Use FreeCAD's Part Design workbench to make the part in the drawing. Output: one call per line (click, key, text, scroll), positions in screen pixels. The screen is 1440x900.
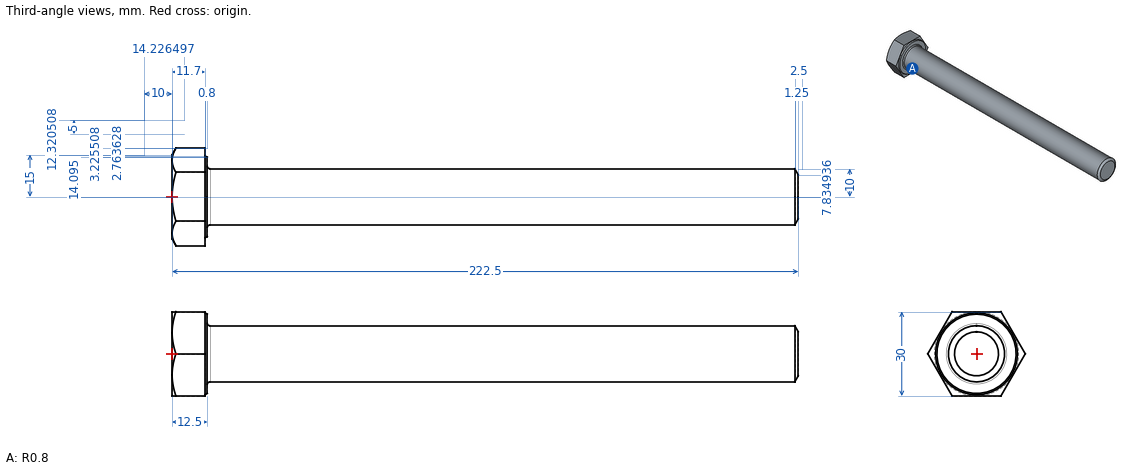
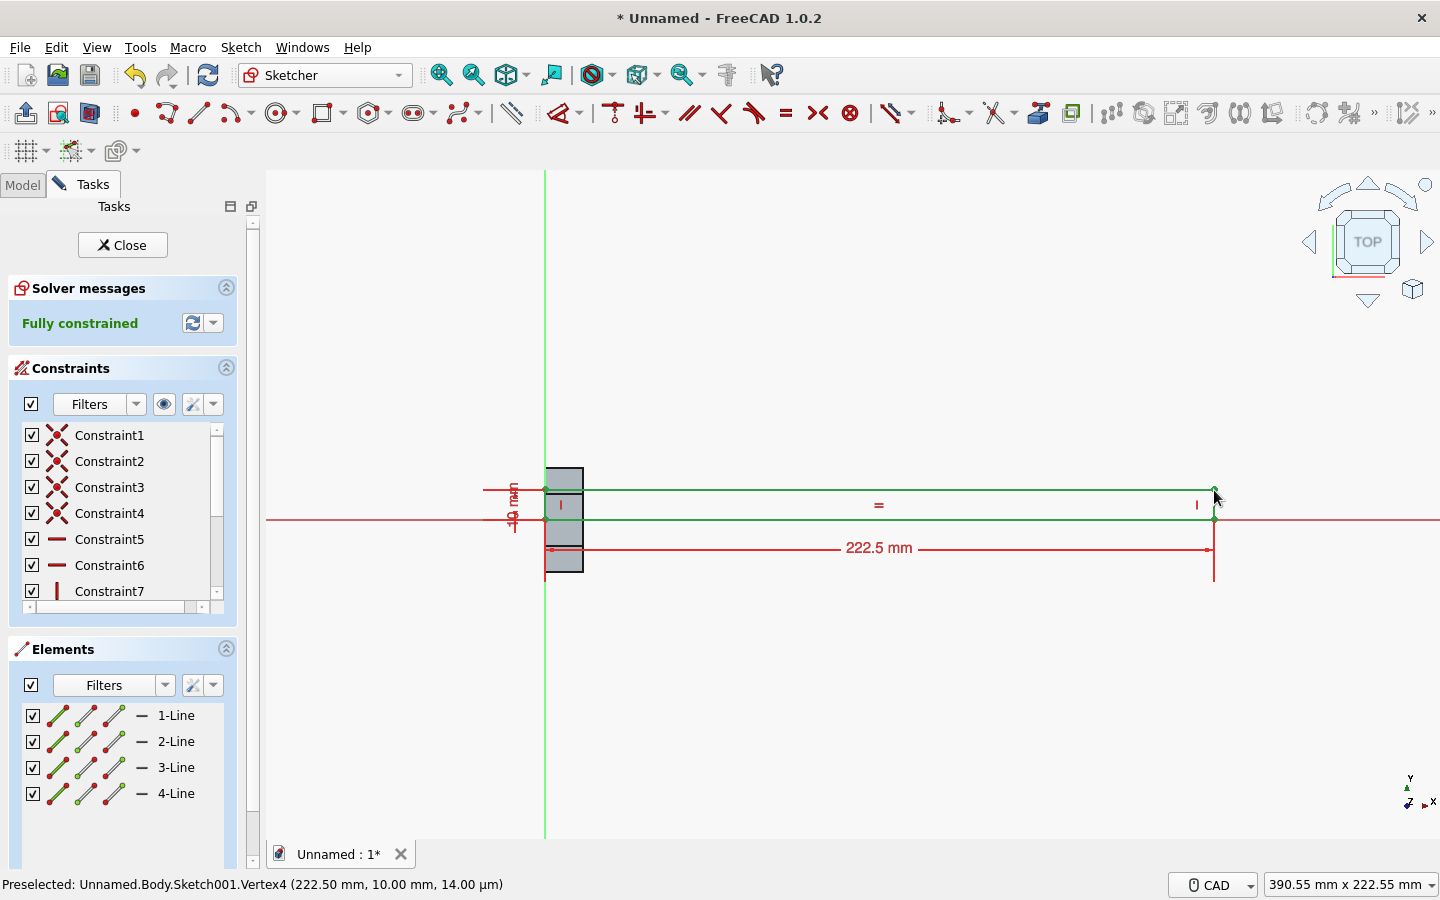
click(123, 245)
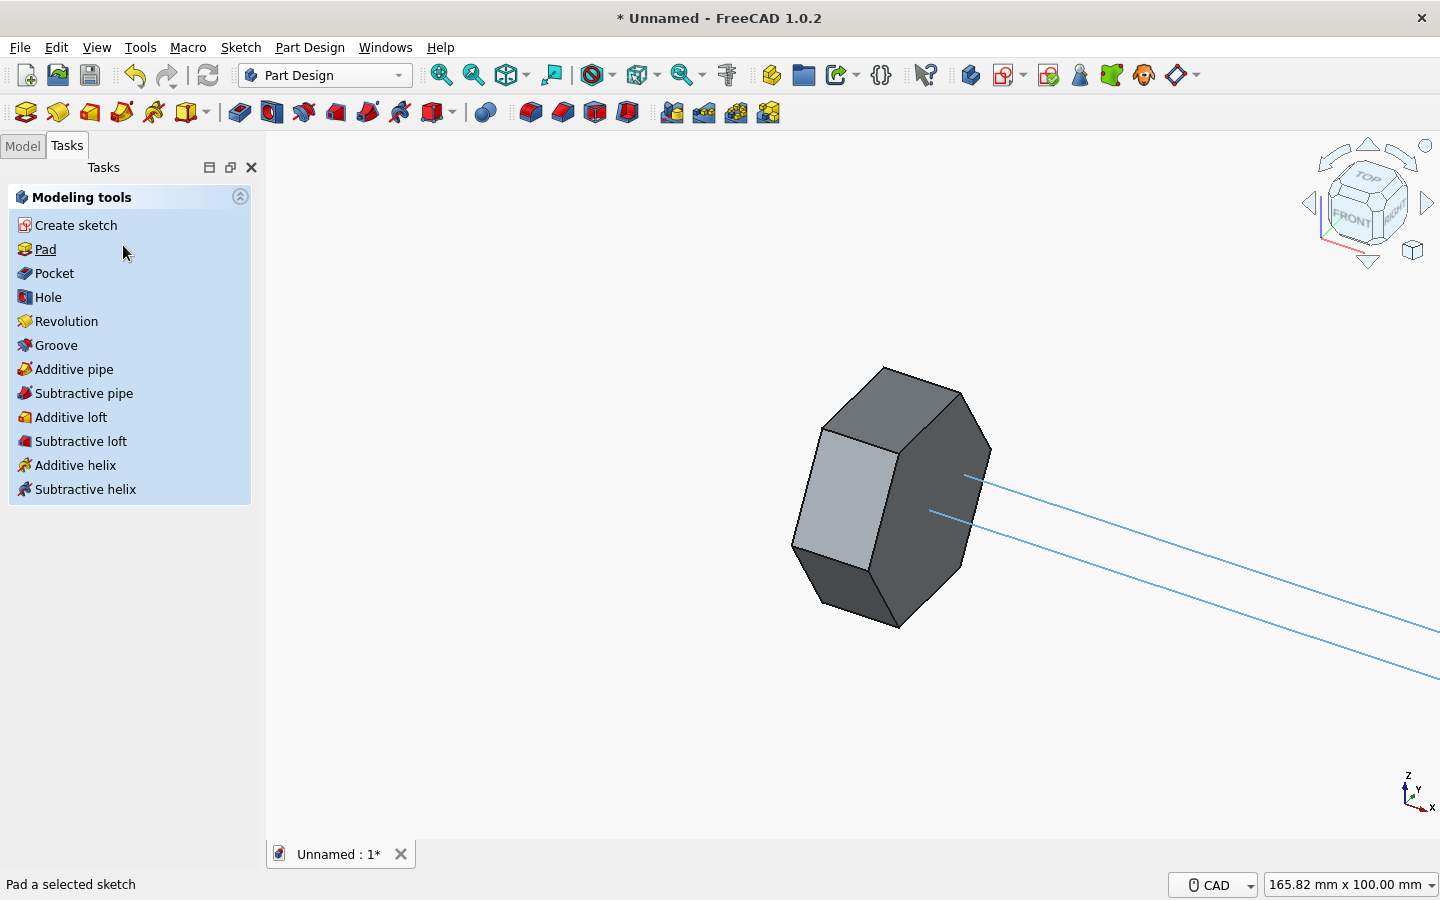
click(58, 112)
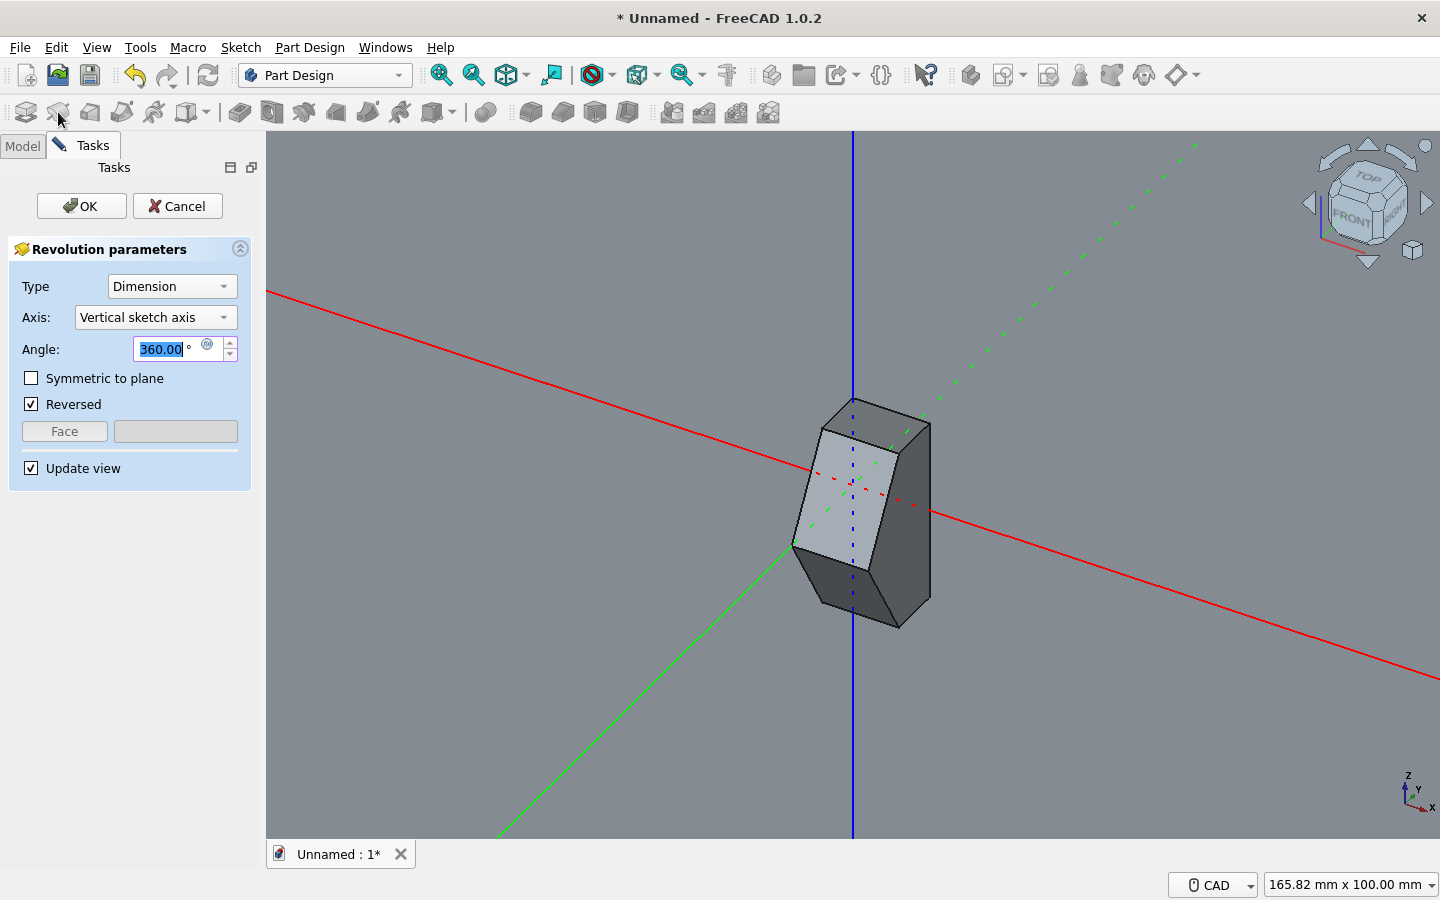
click(156, 318)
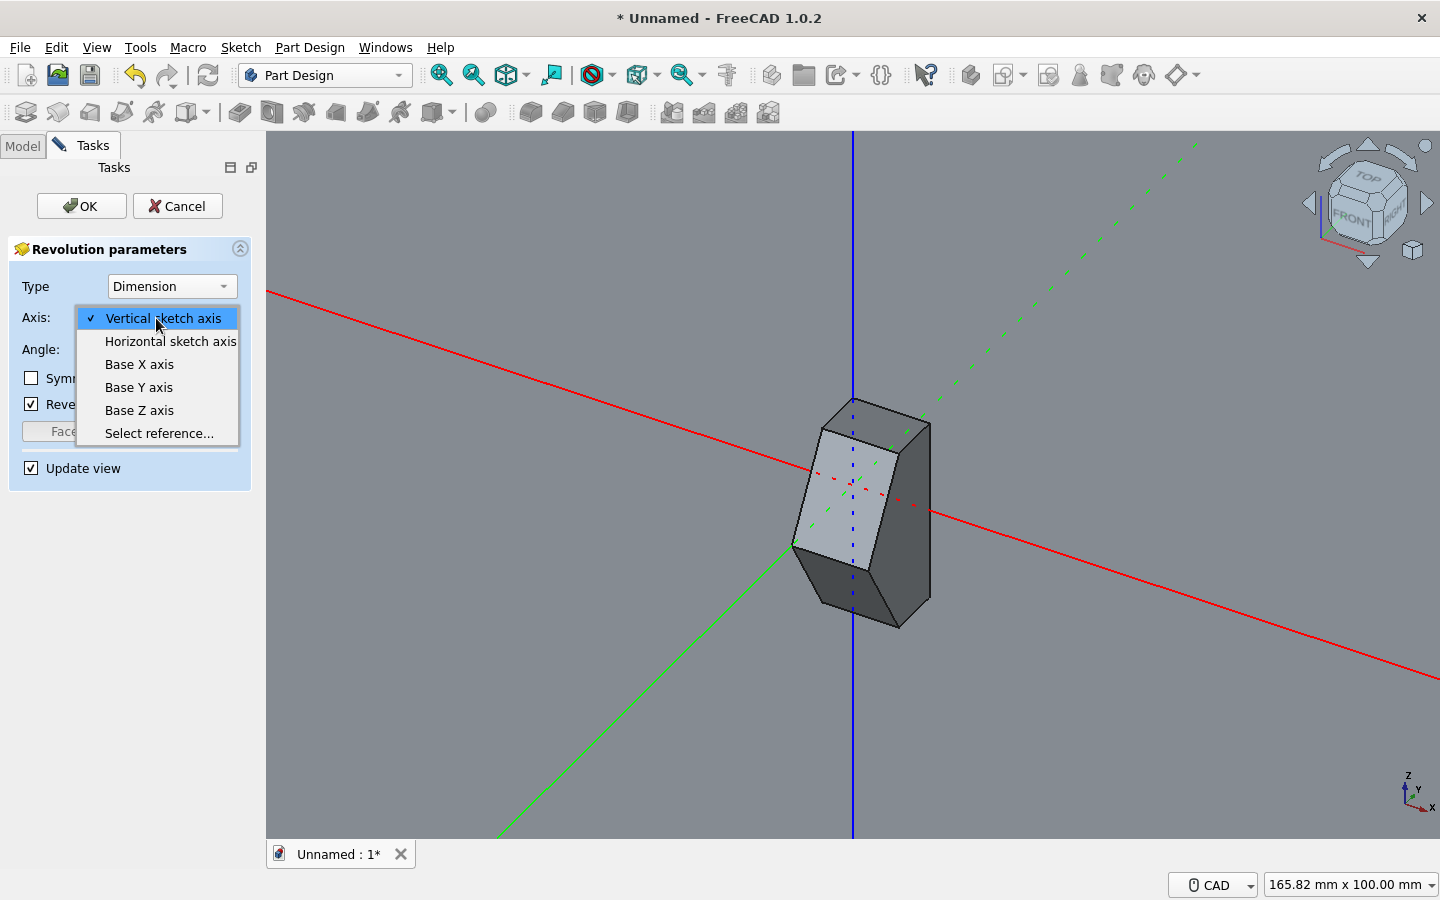
click(156, 342)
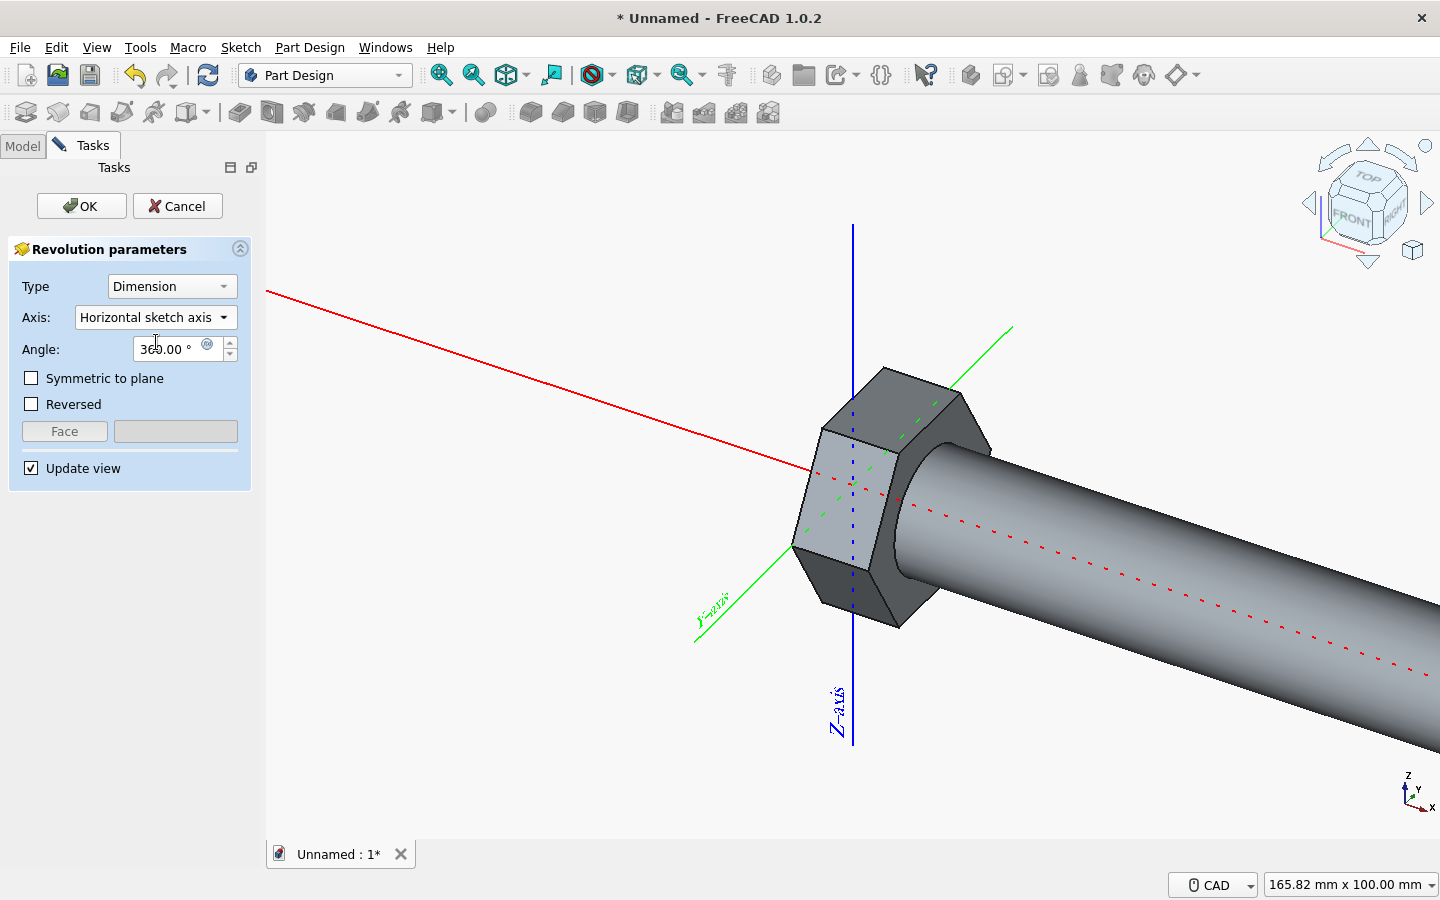
click(82, 206)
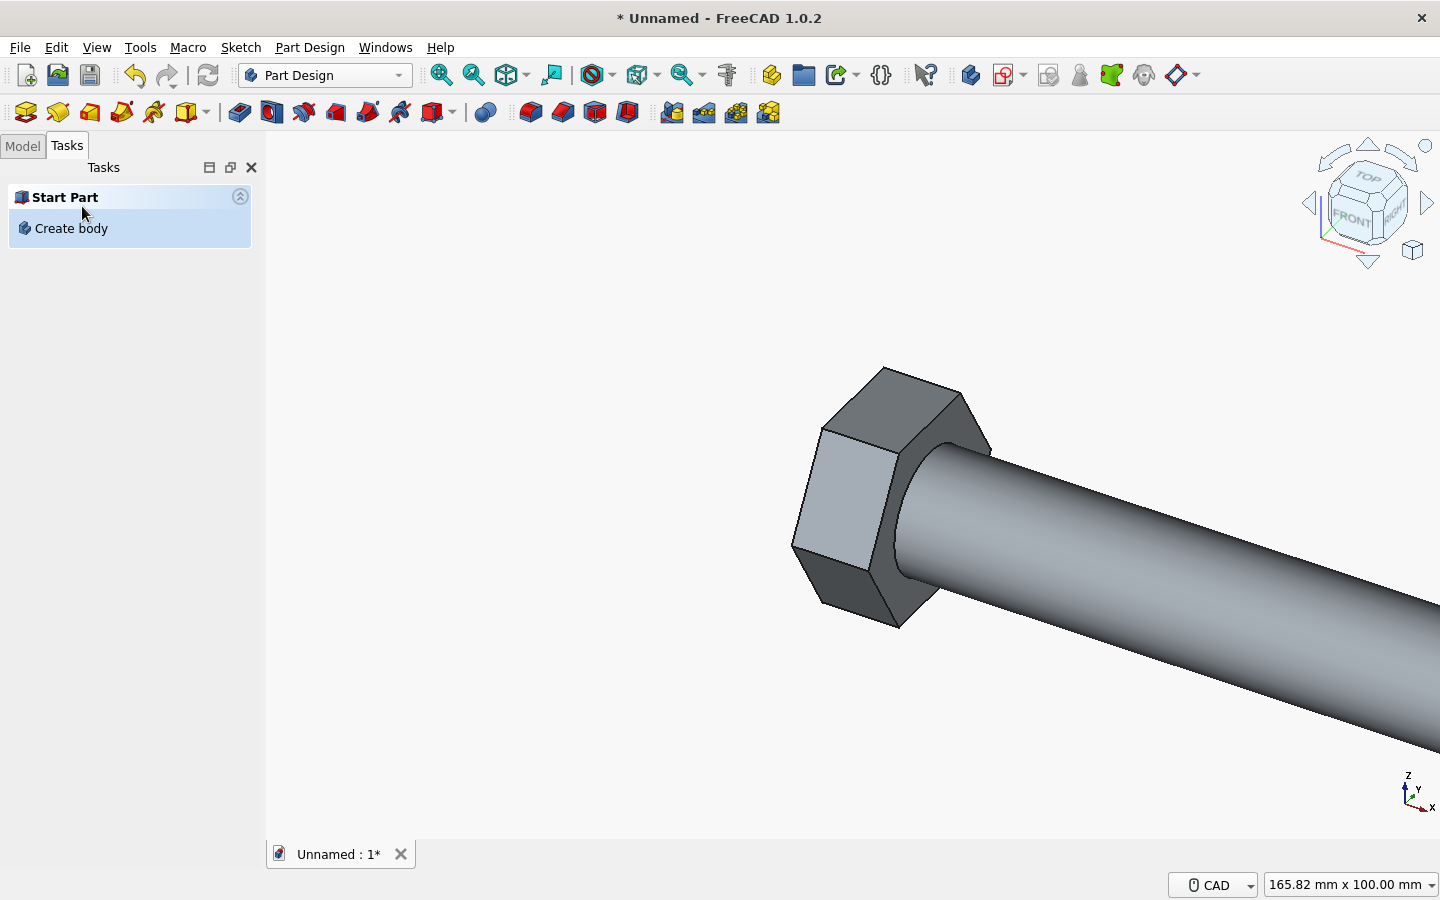
click(442, 76)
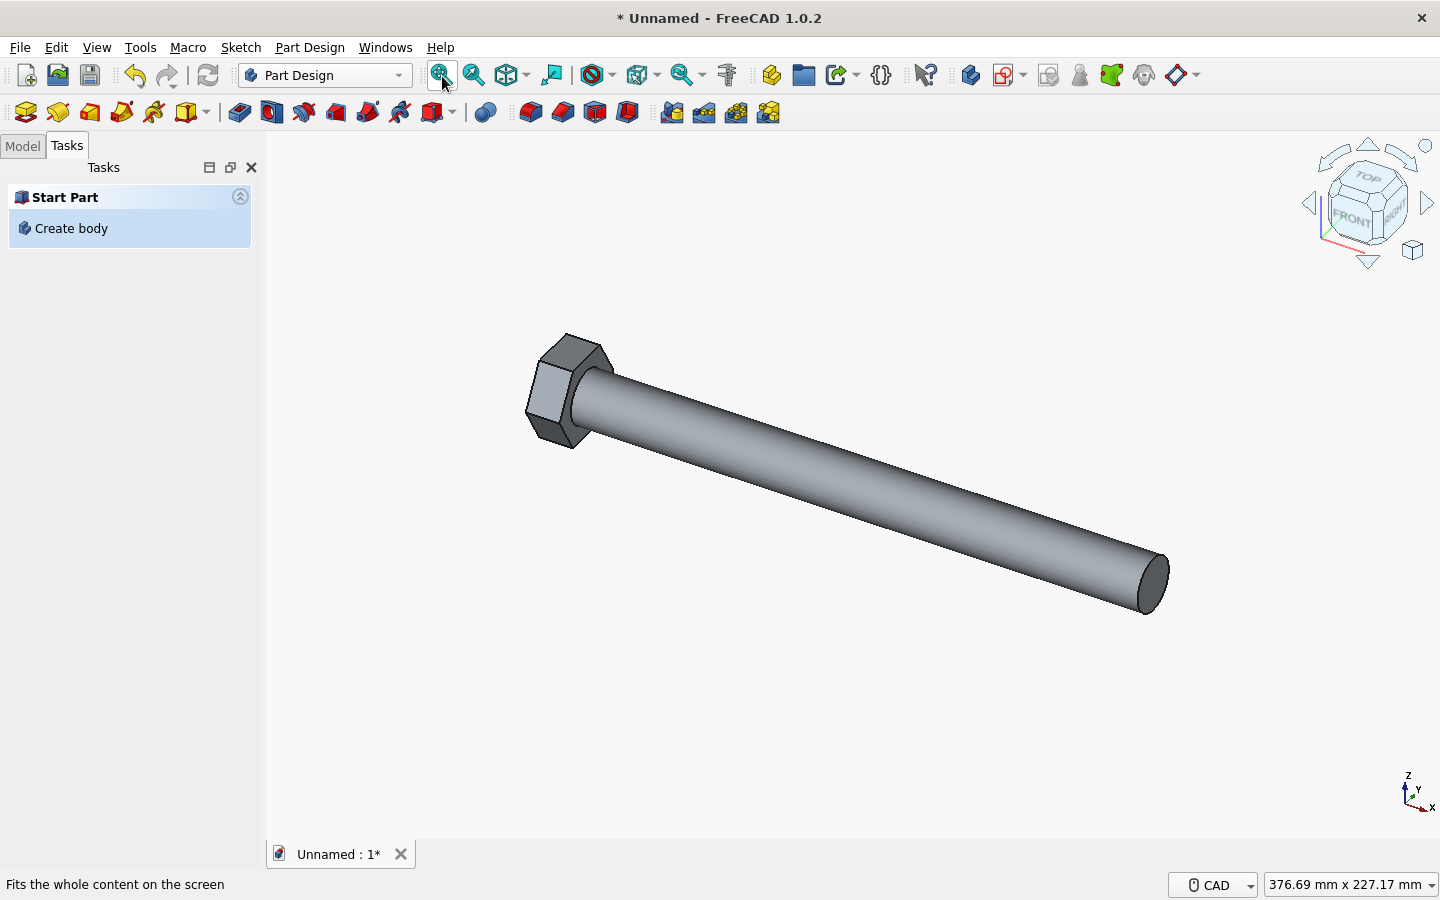
click(1004, 76)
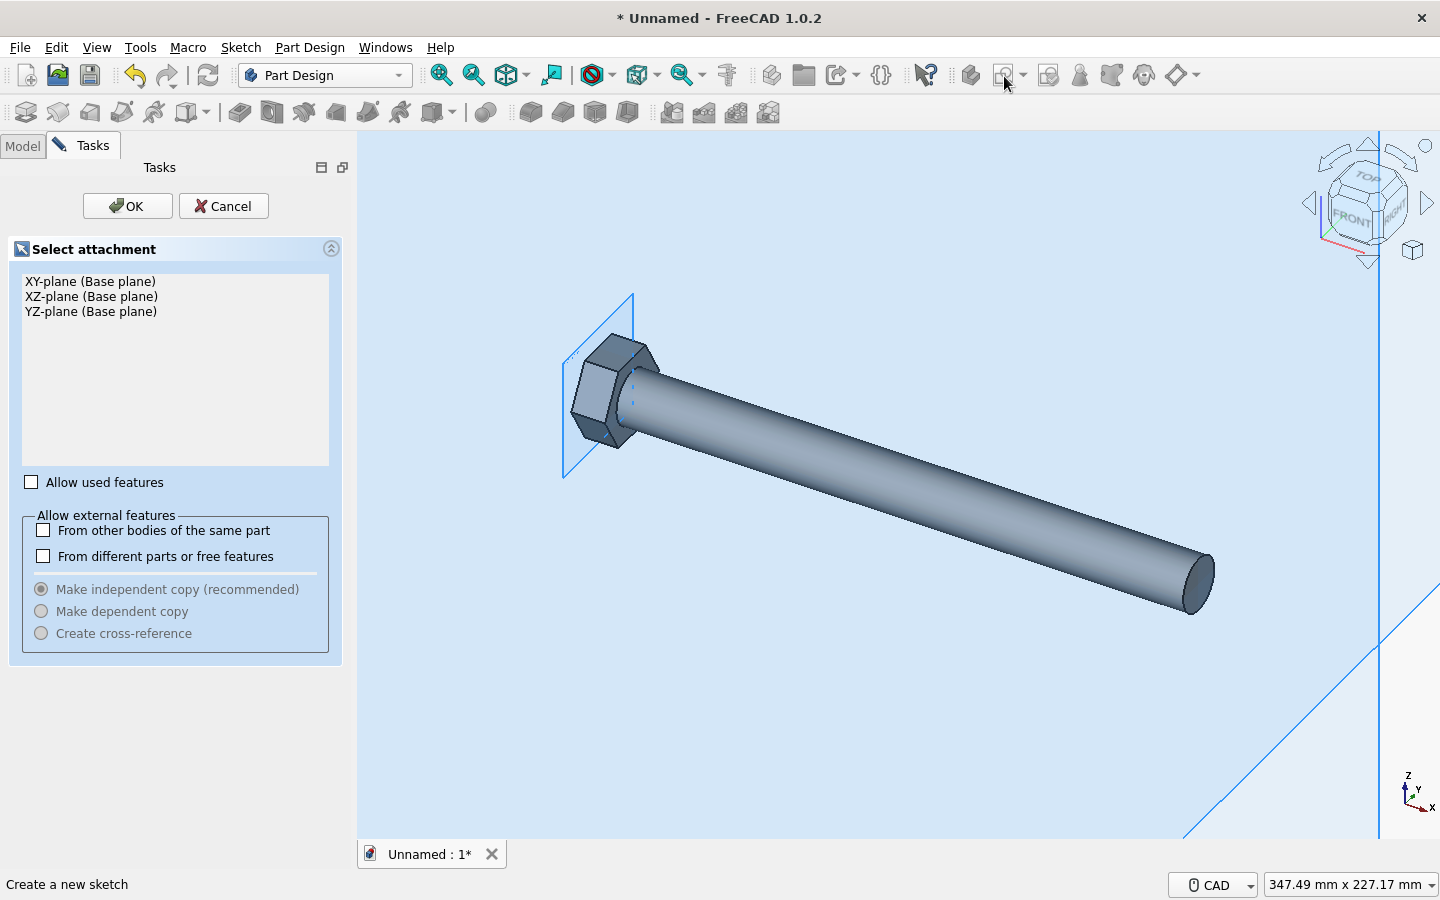
click(82, 282)